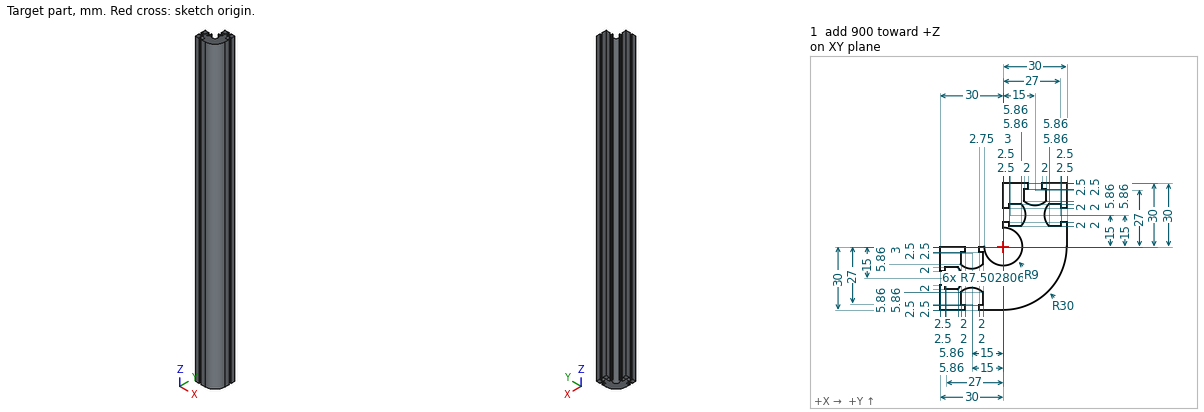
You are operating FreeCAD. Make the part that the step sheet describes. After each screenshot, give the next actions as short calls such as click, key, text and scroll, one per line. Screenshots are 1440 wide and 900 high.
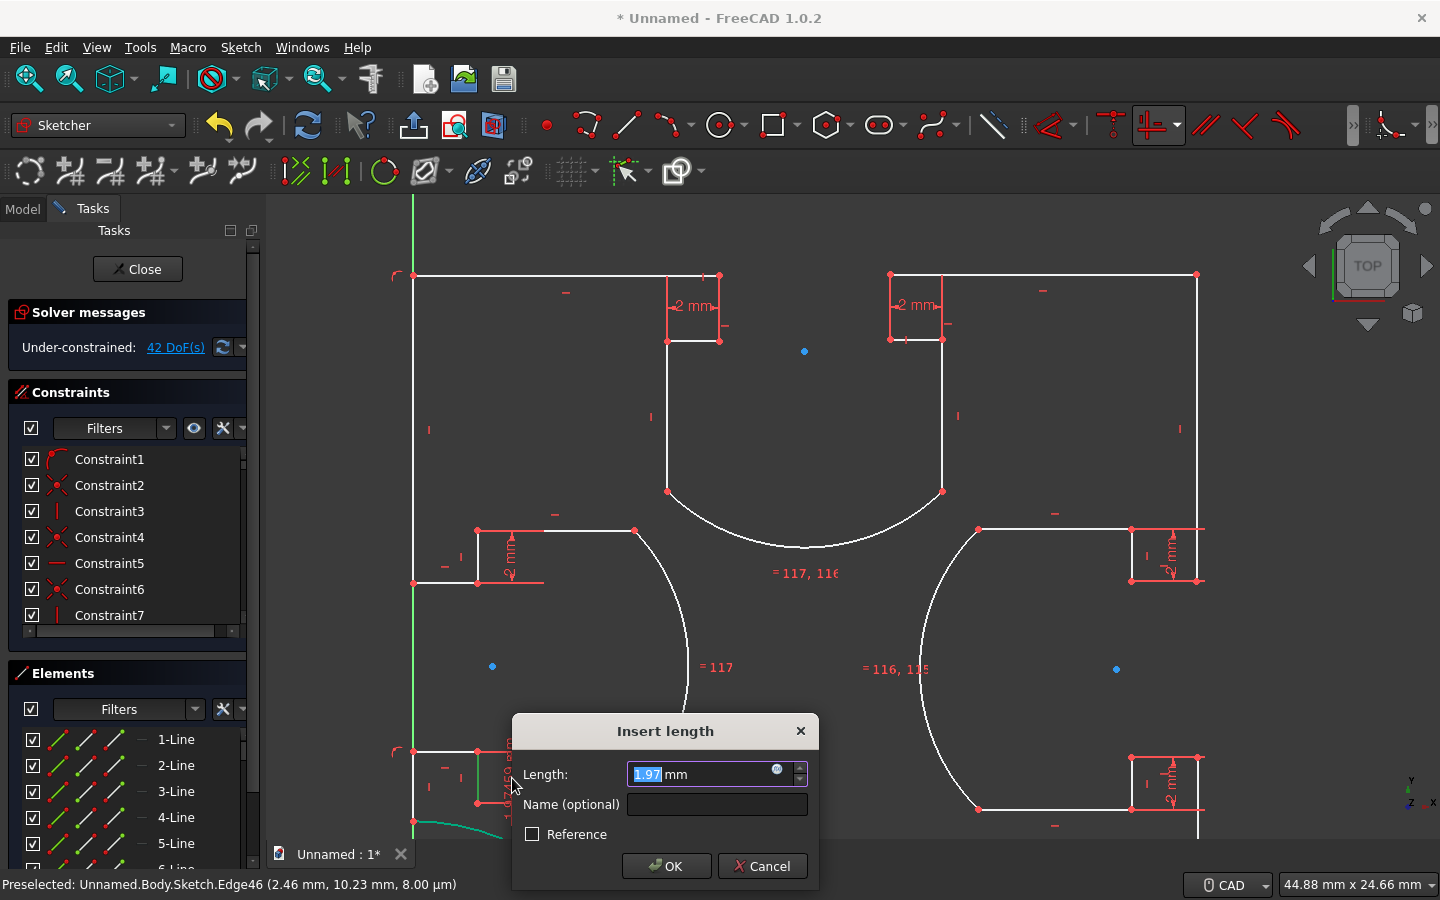
text(2)
key(Return)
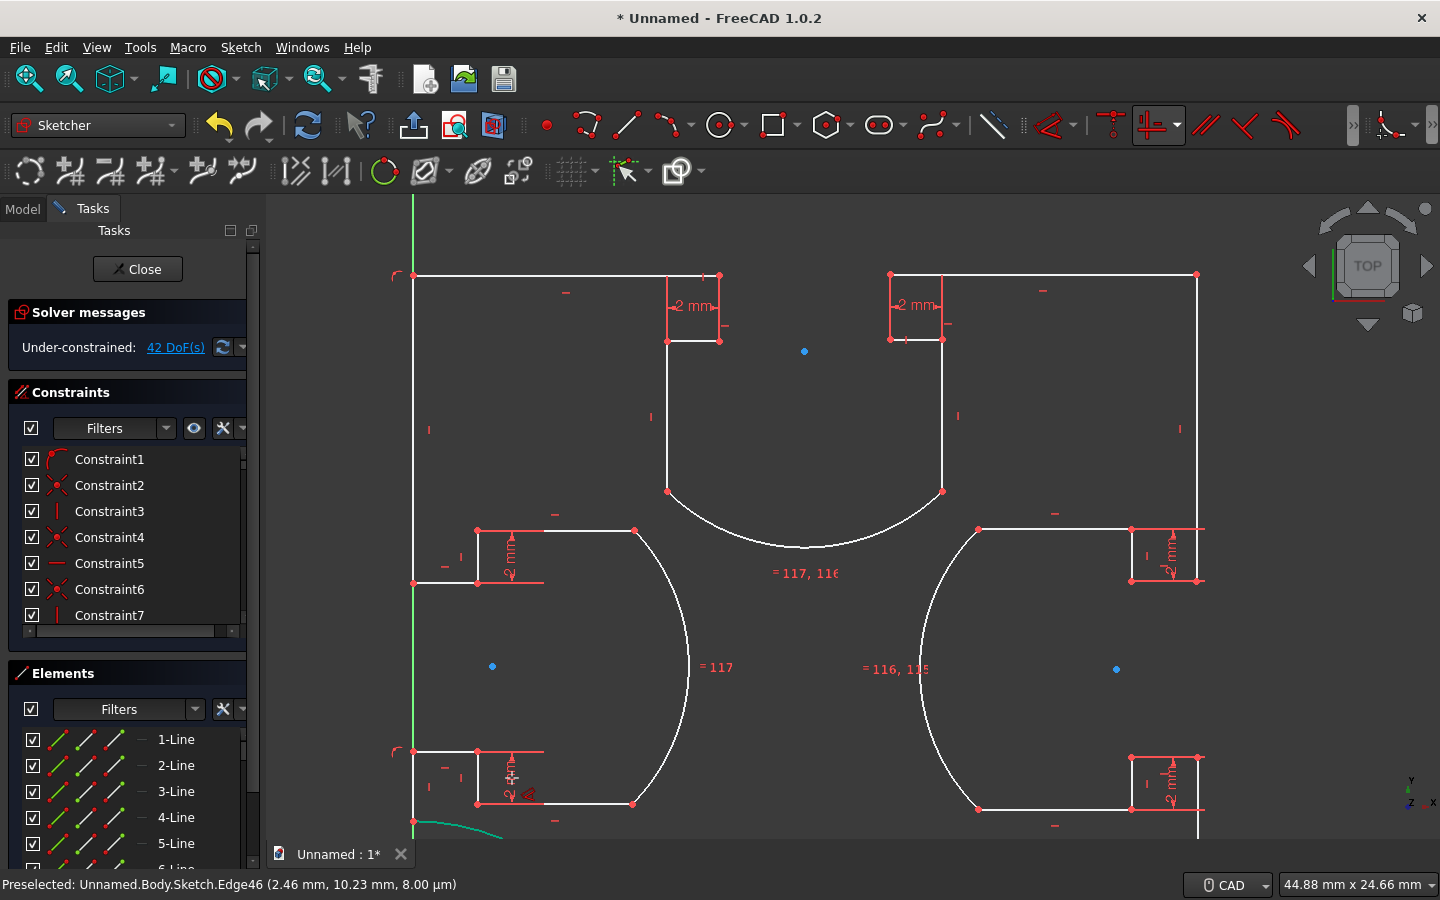
scroll(906, 340, down, 7)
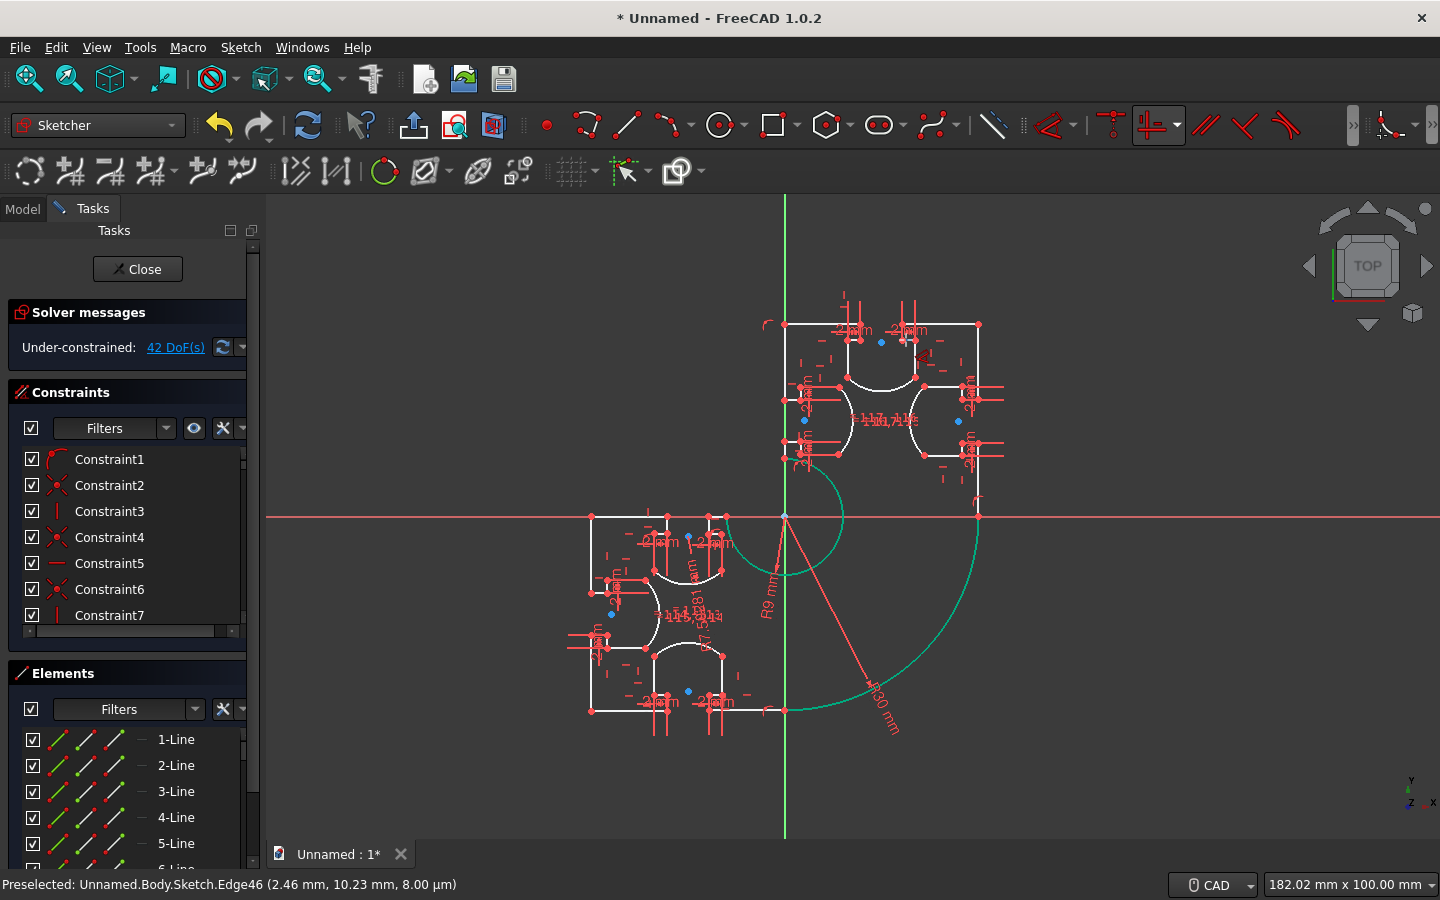
scroll(688, 536, up, 4)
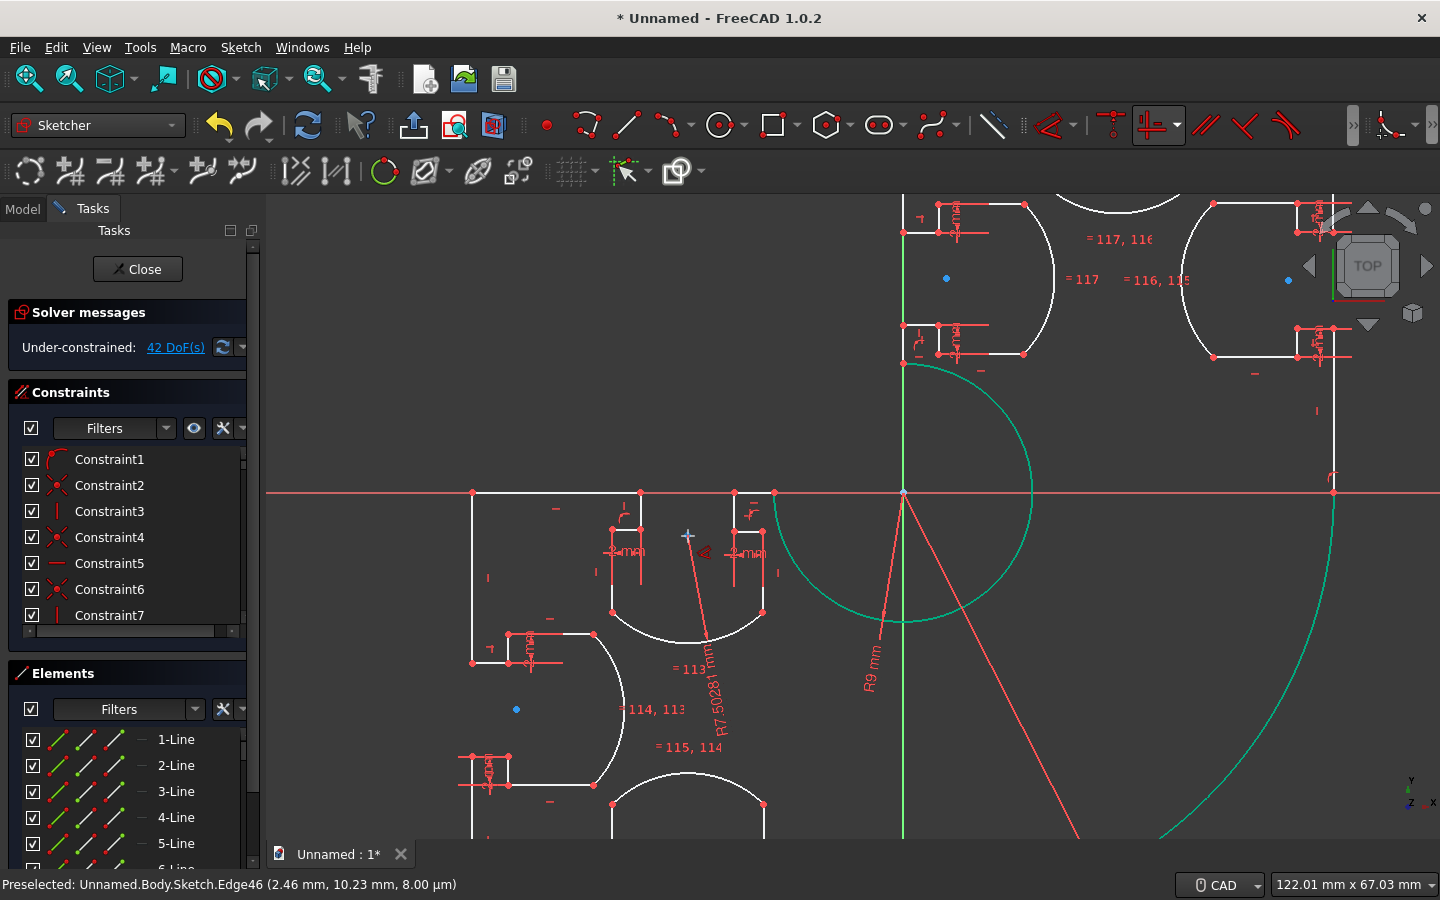
click(688, 536)
click(937, 514)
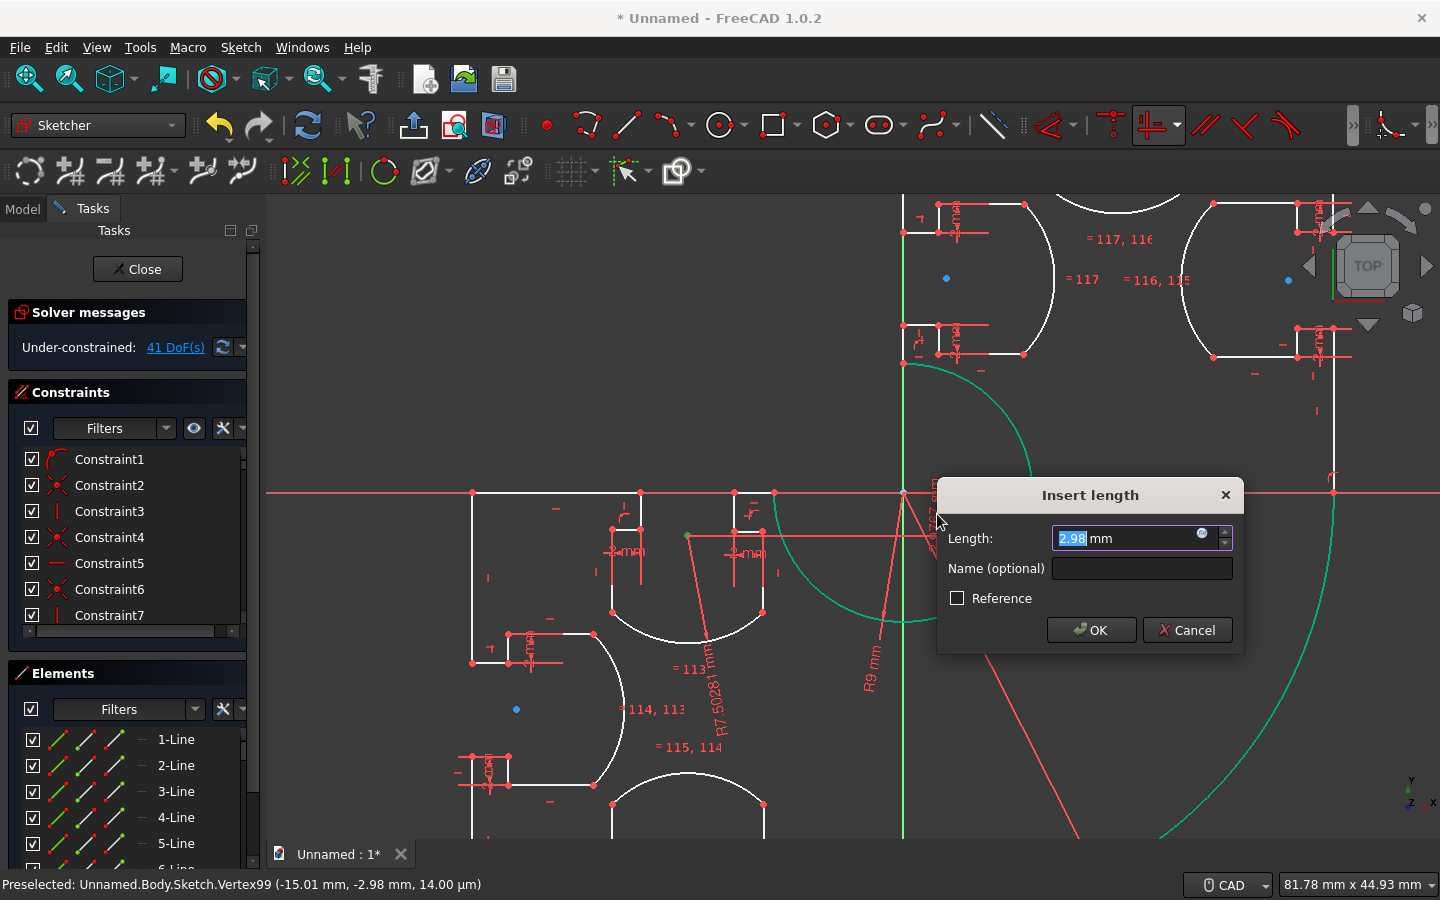
text(3)
key(Return)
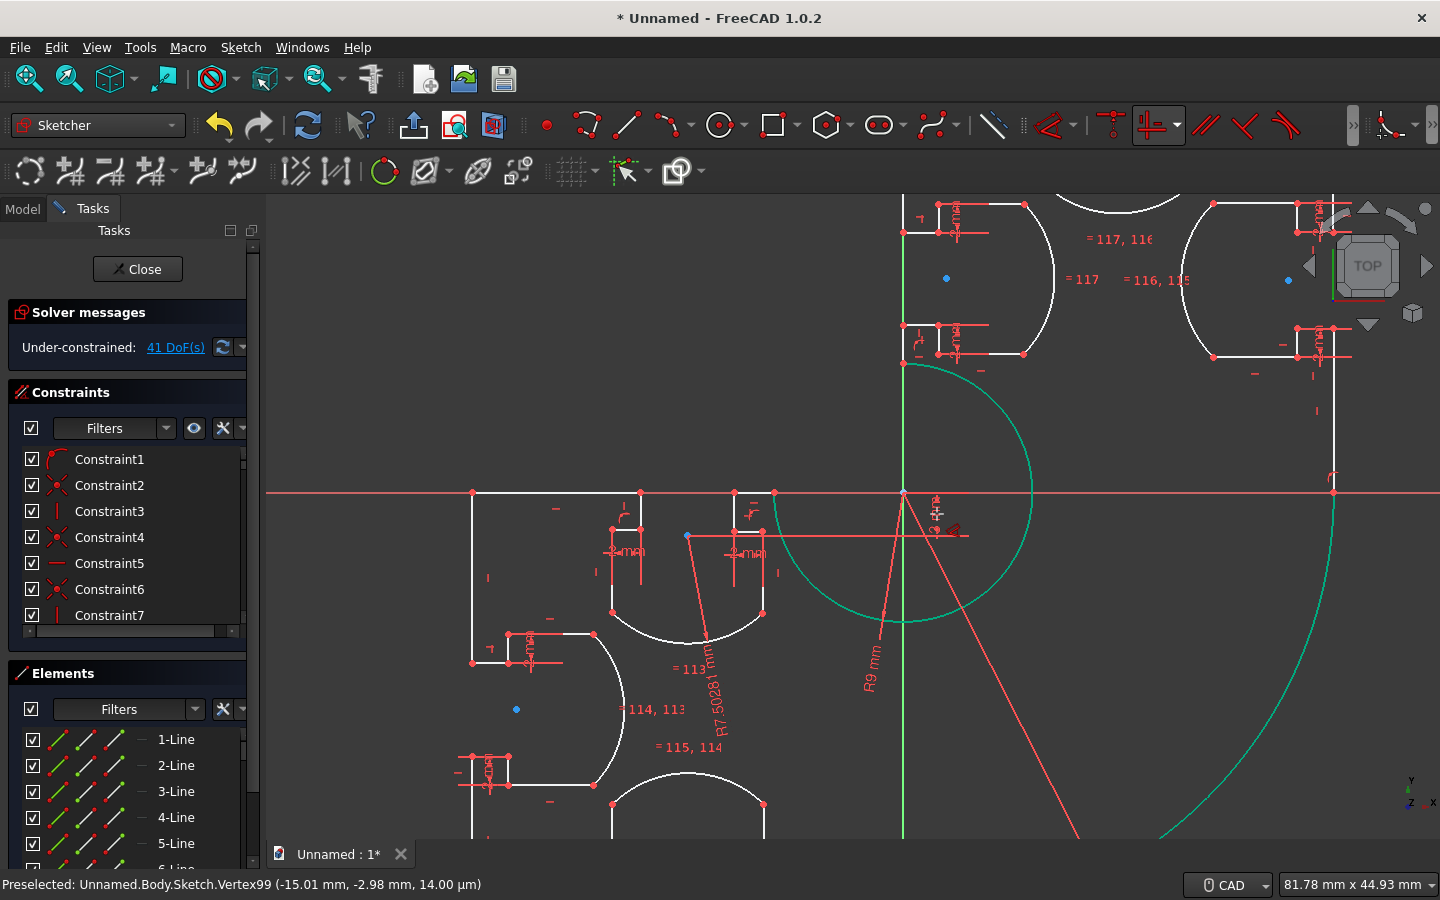
click(947, 279)
click(925, 551)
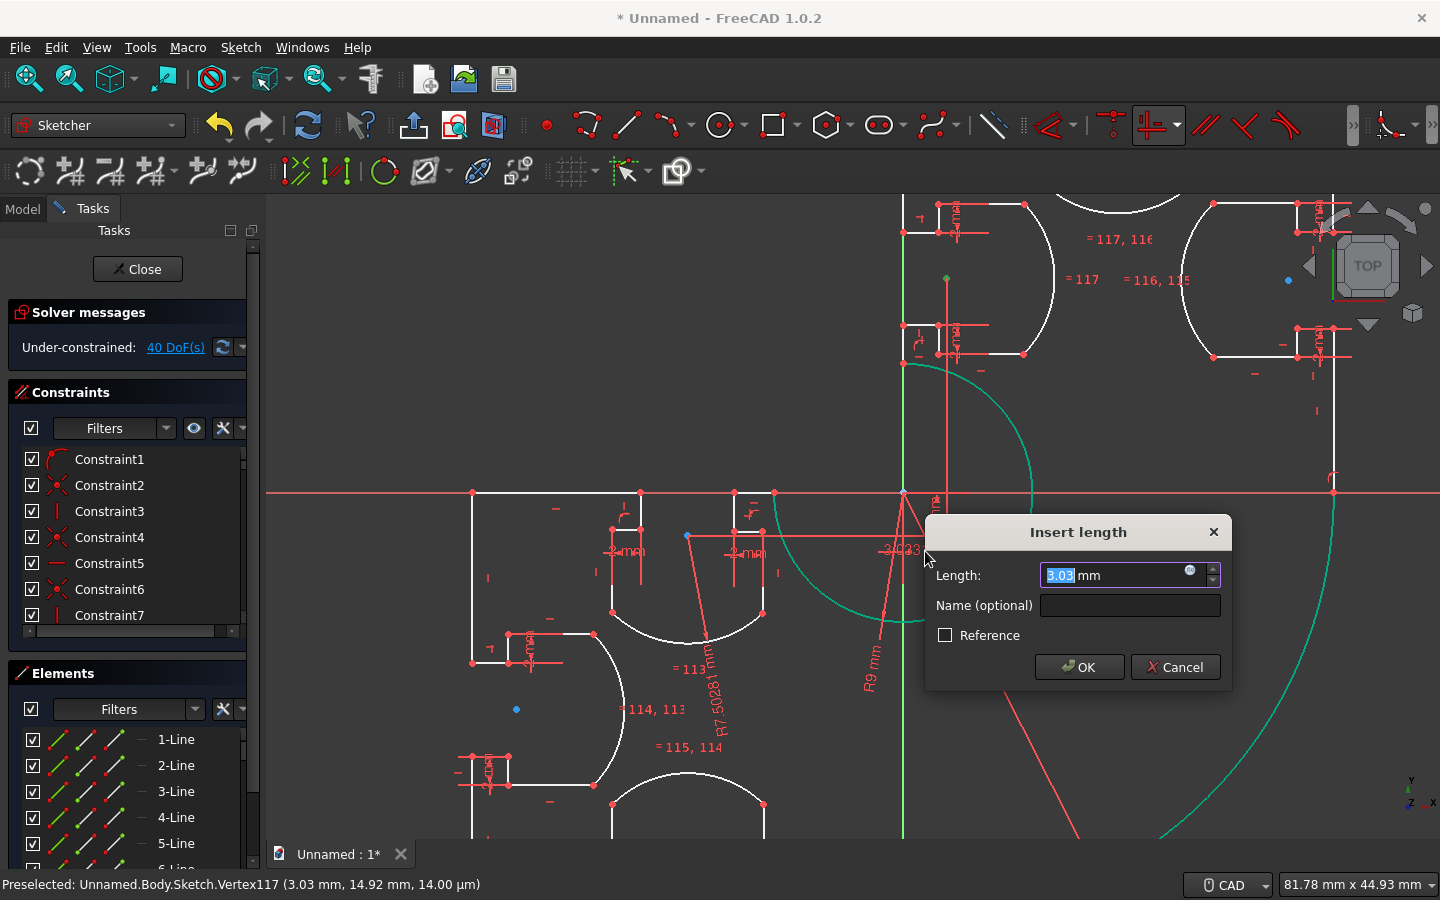
text(3)
key(Return)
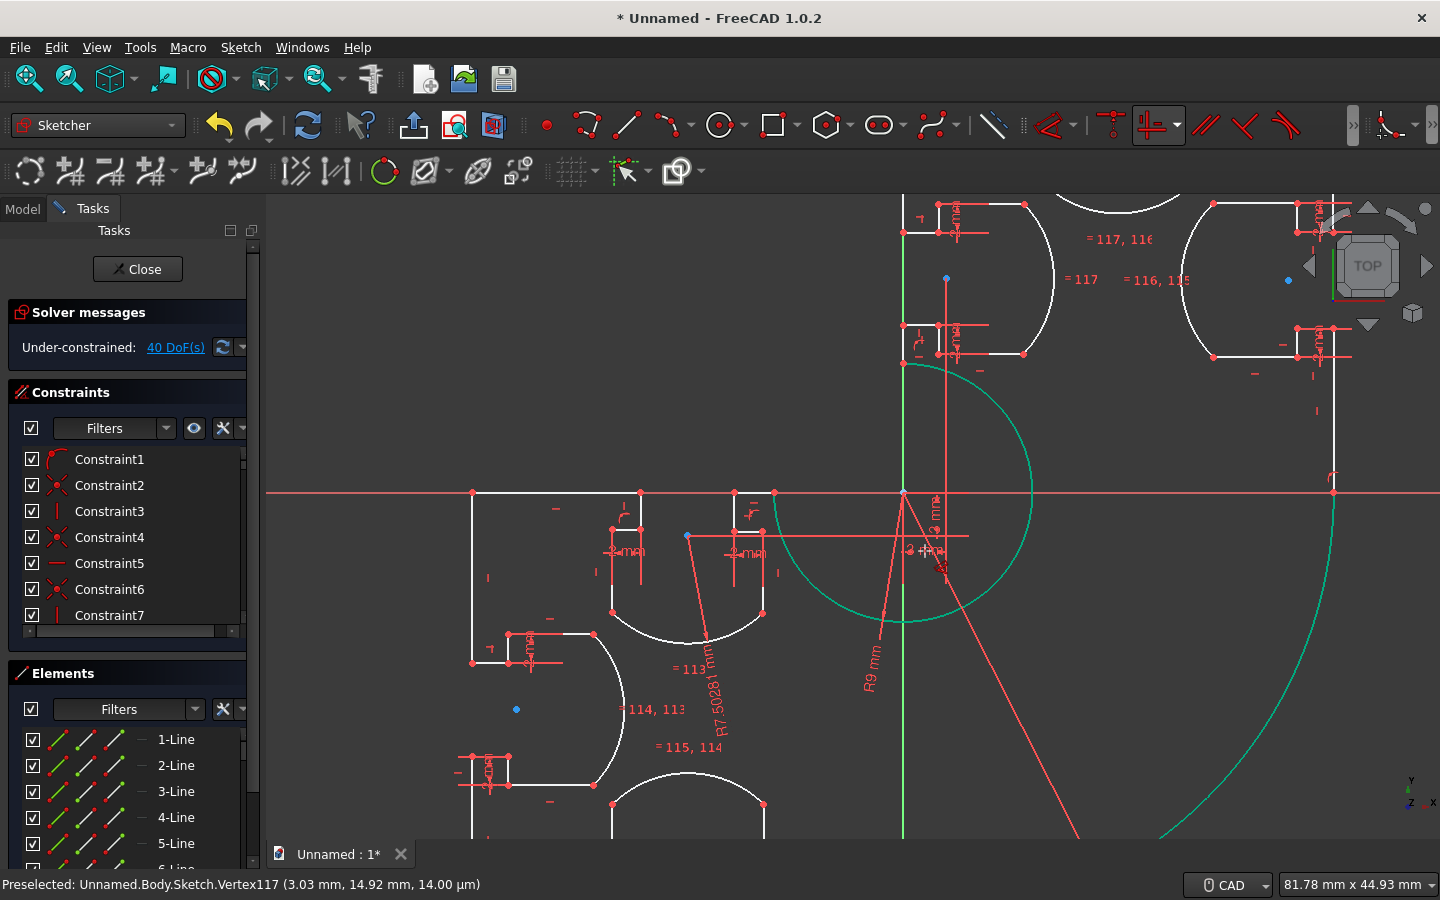
click(734, 505)
click(700, 512)